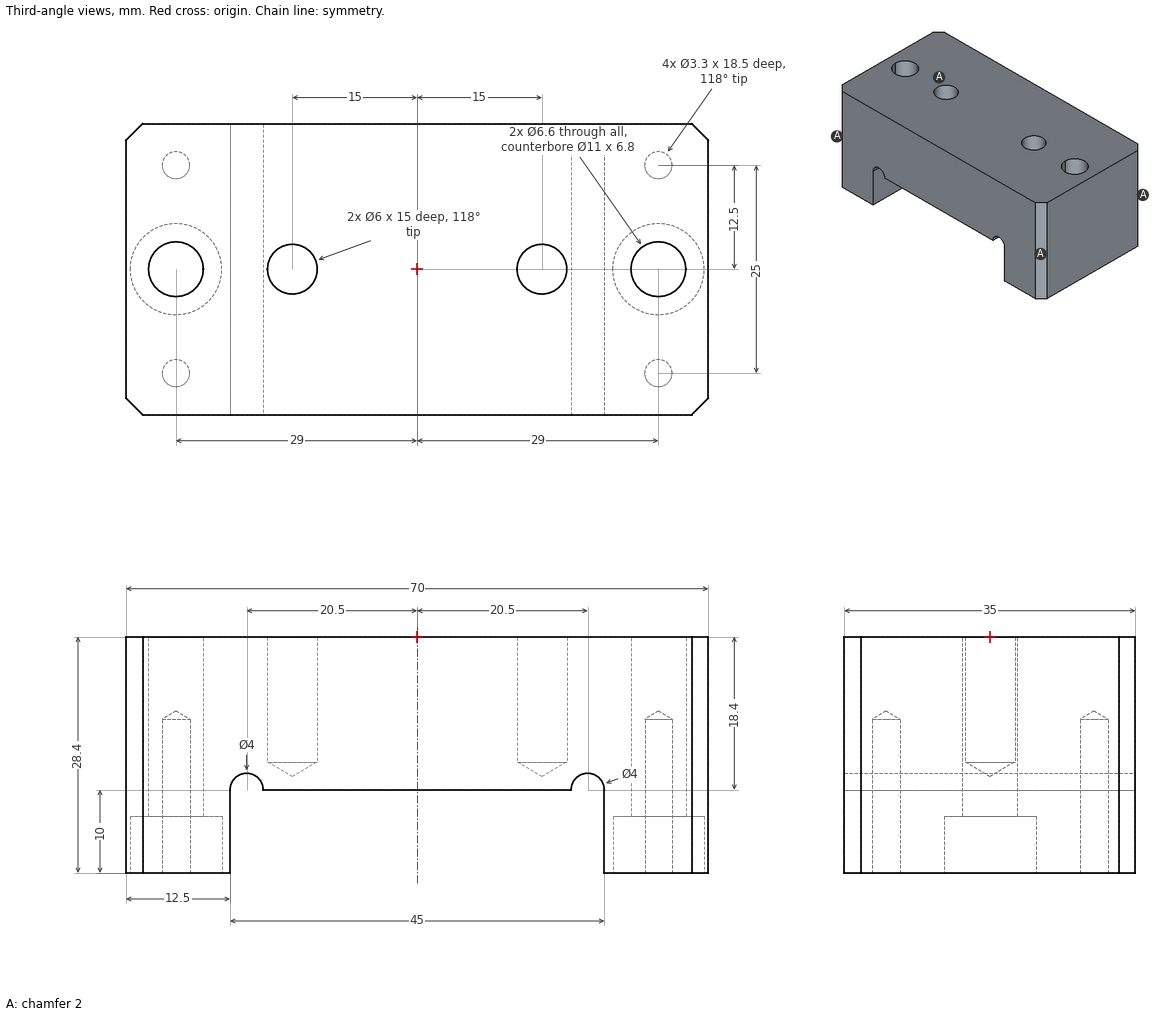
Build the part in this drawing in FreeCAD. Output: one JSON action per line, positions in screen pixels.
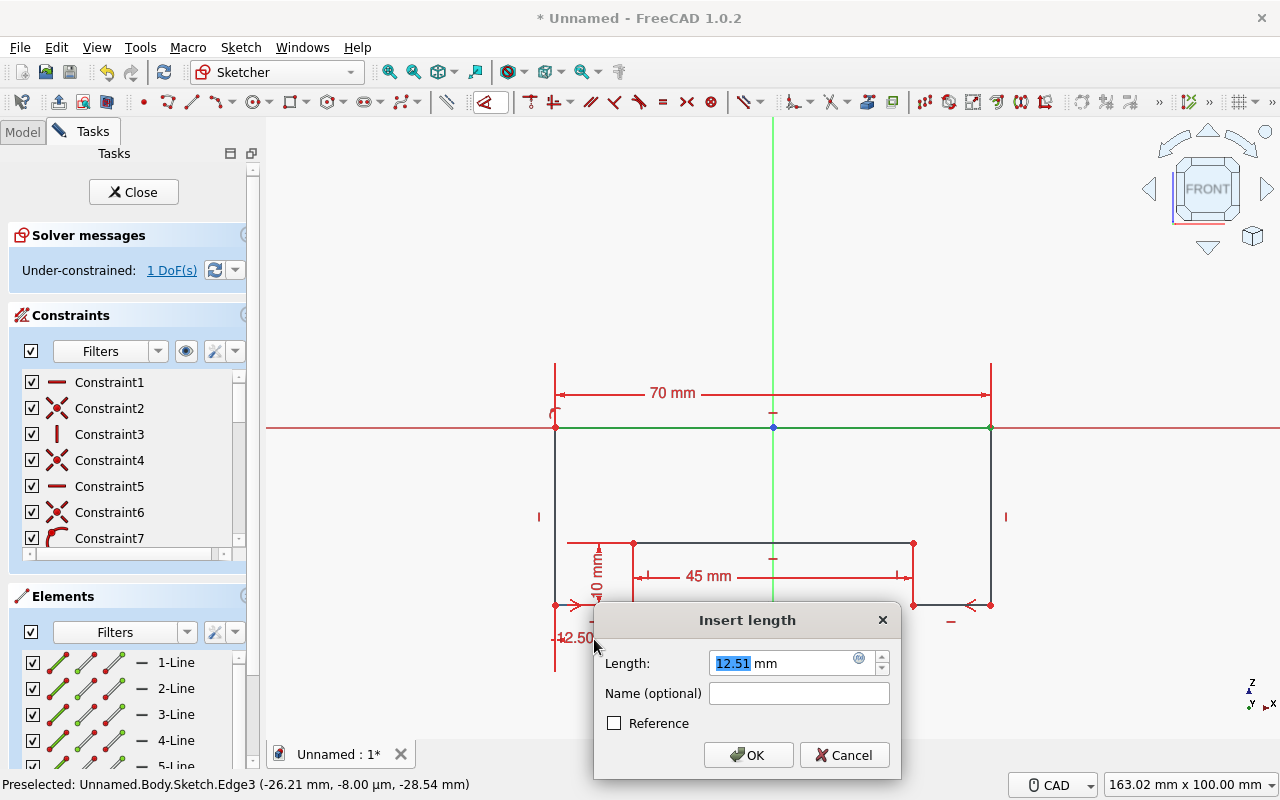
{"action": "type", "text": "12.5"}
{"action": "key", "text": "Return"}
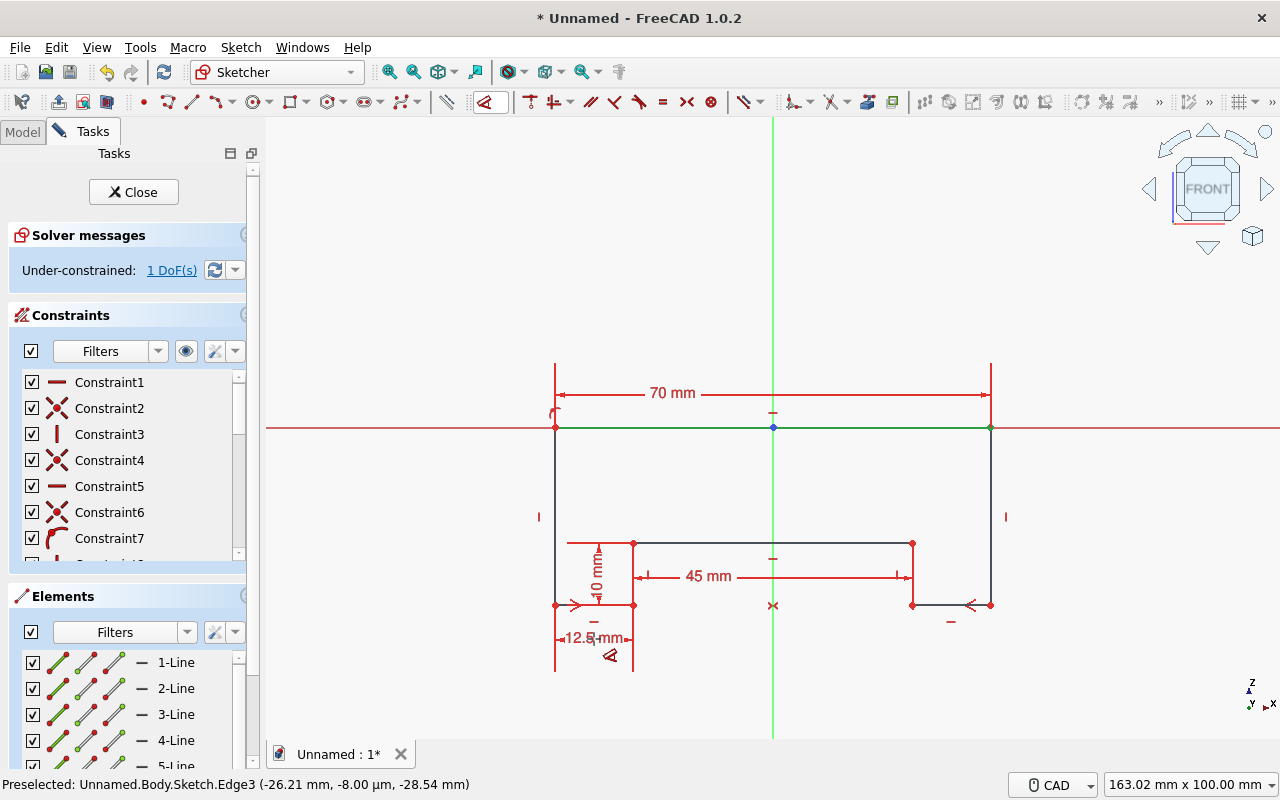
{"action": "left_click", "coordinate": [555, 552]}
{"action": "left_click", "coordinate": [521, 517]}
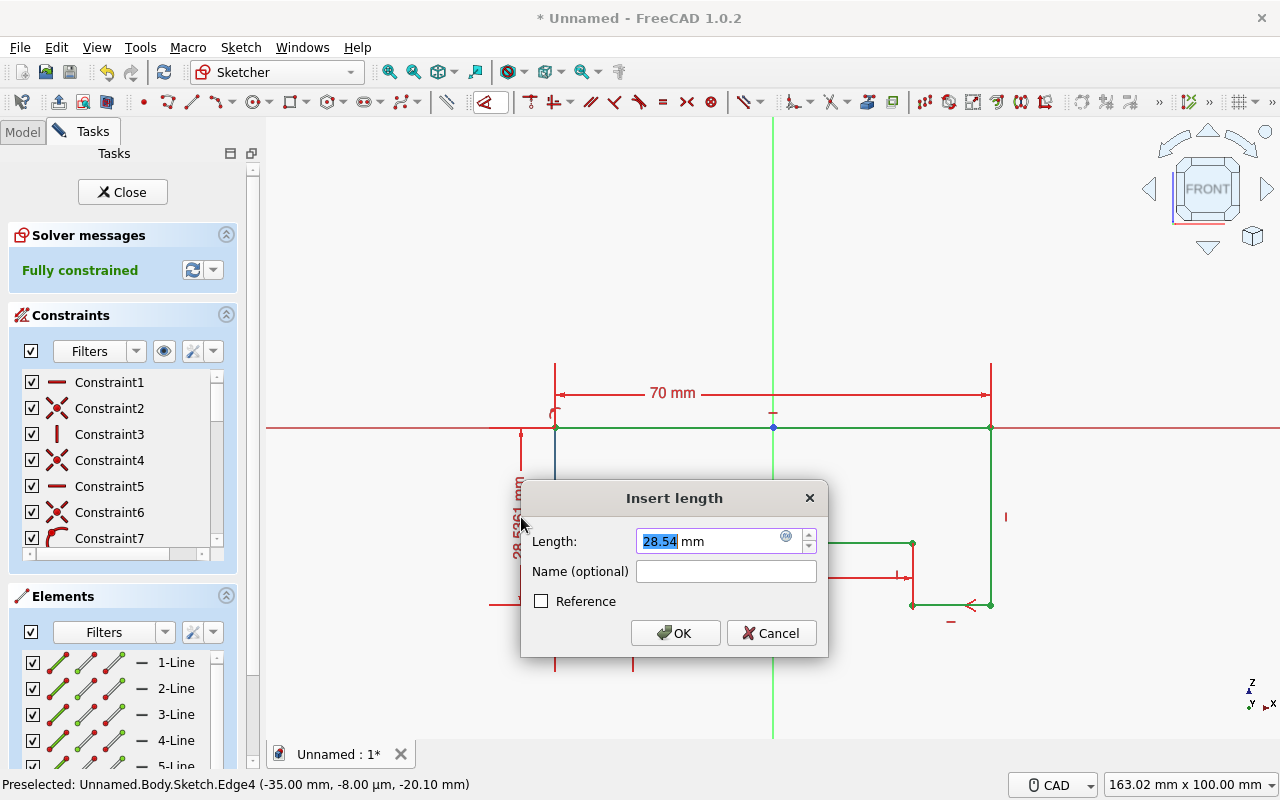
{"action": "type", "text": "28.4"}
{"action": "key", "text": "Return"}
{"action": "key", "text": "Escape"}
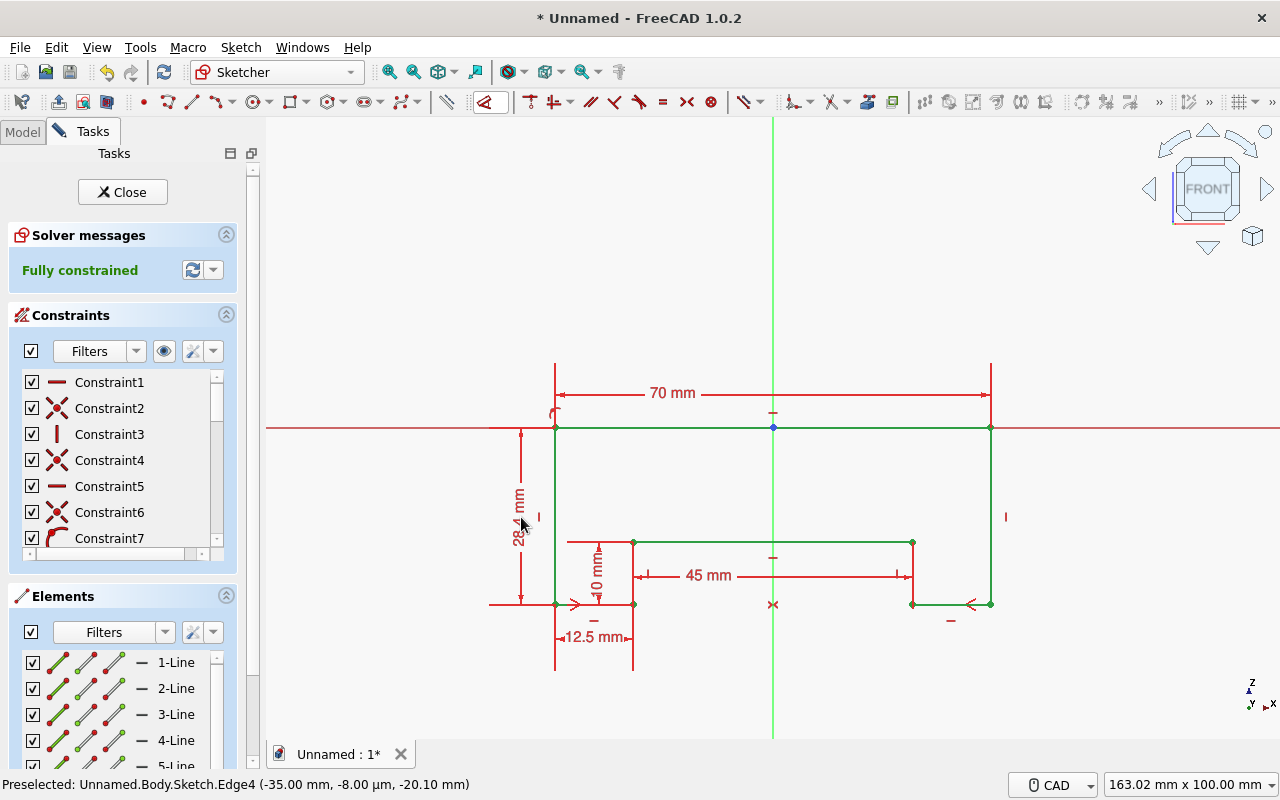
{"action": "left_click", "coordinate": [123, 192]}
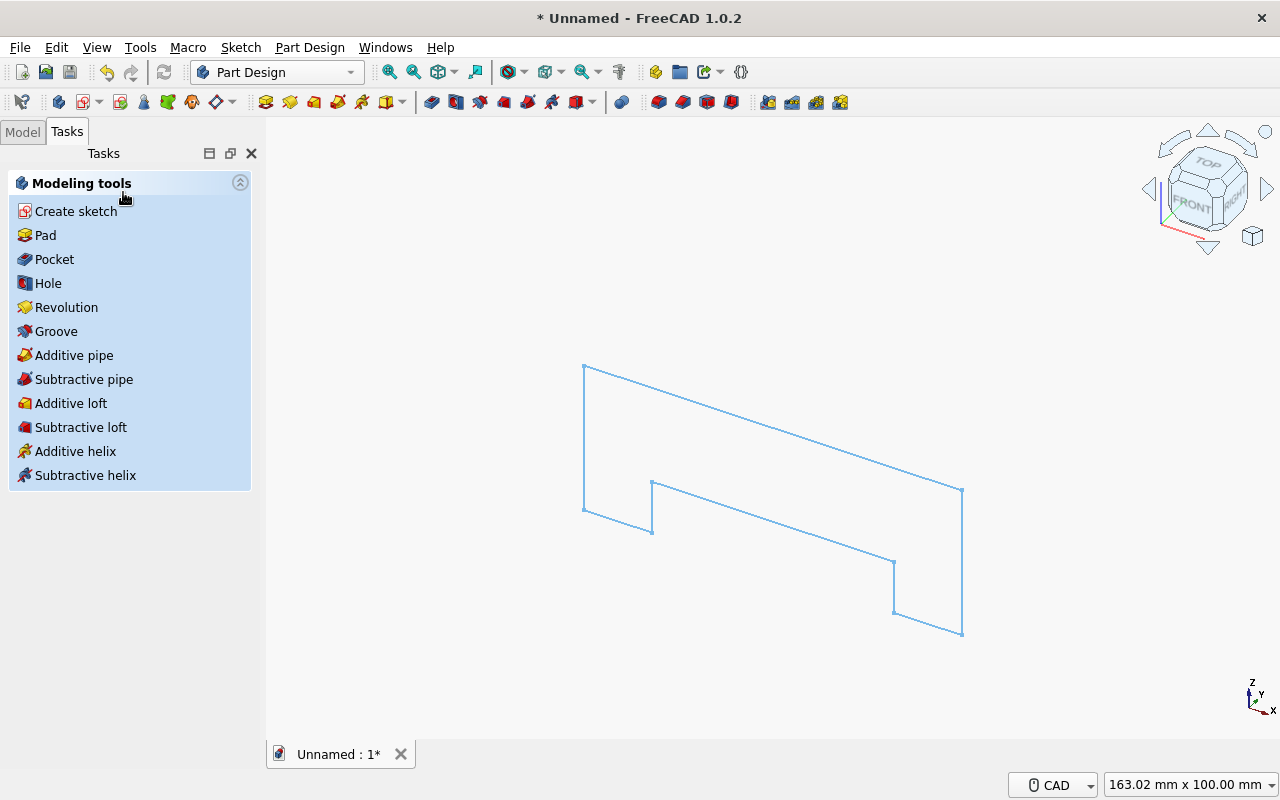
{"action": "left_click", "coordinate": [266, 102]}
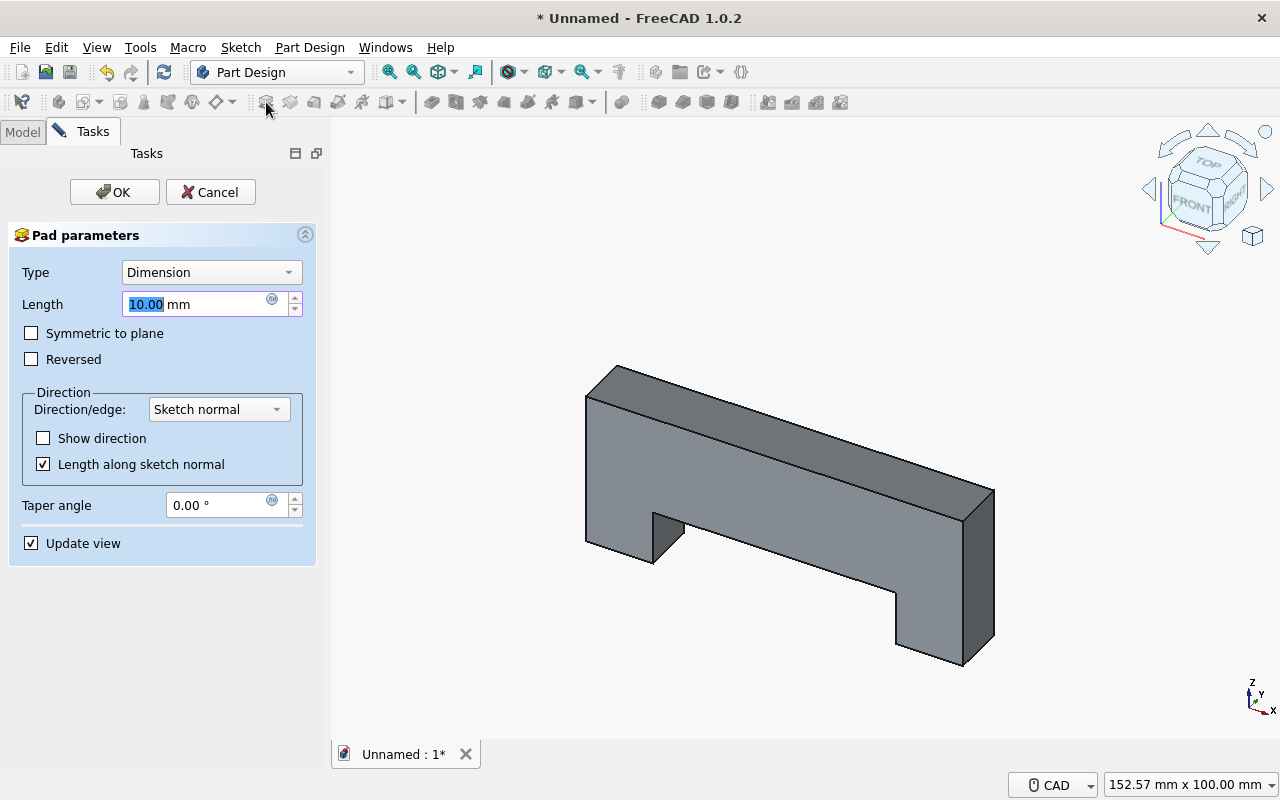
{"action": "type", "text": "35"}
{"action": "key", "text": "Tab"}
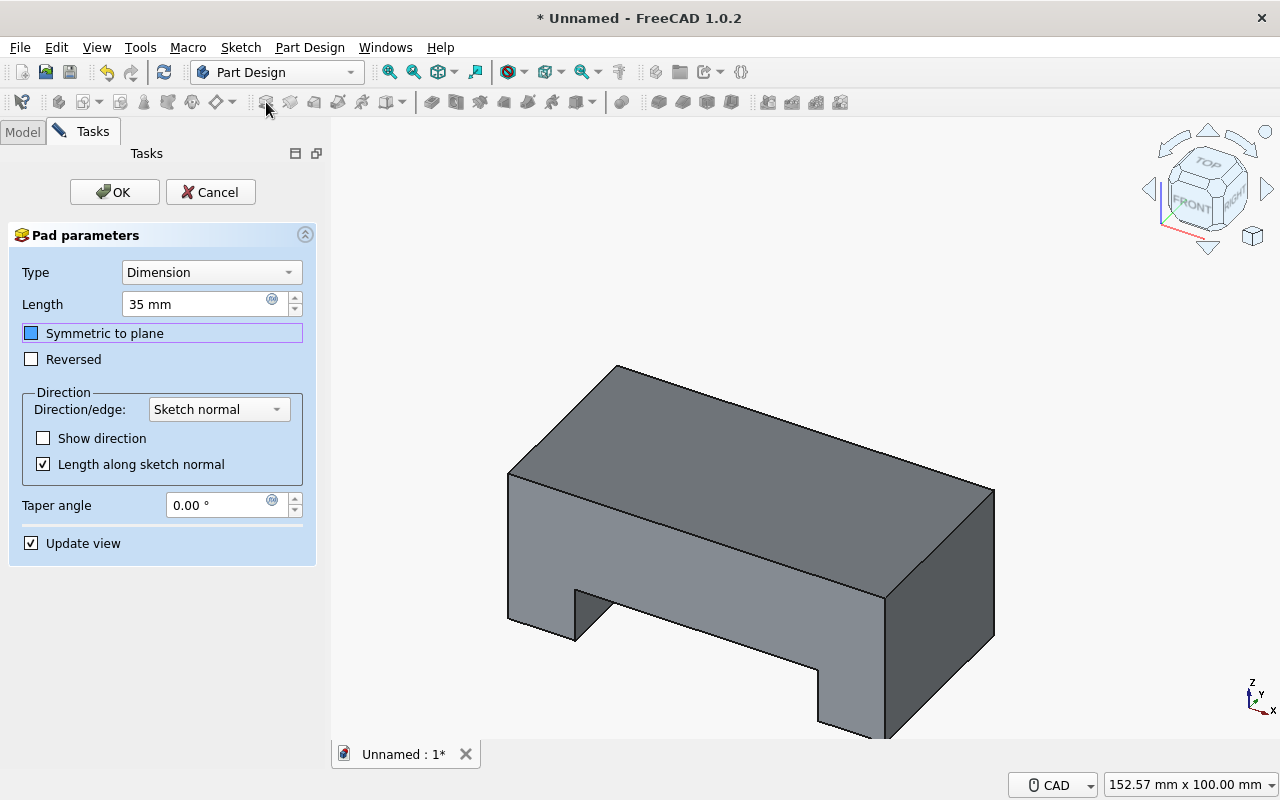
{"action": "left_click", "coordinate": [30, 333]}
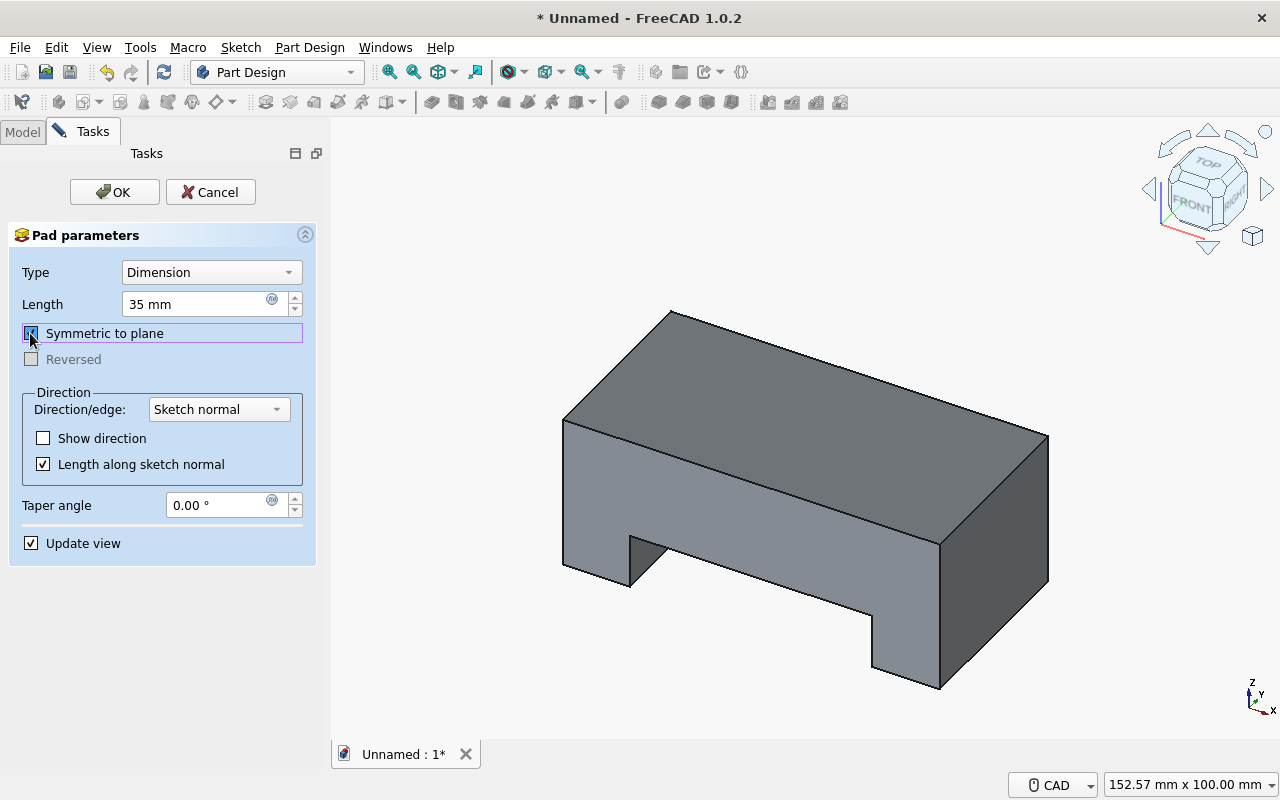
{"action": "left_click", "coordinate": [115, 192]}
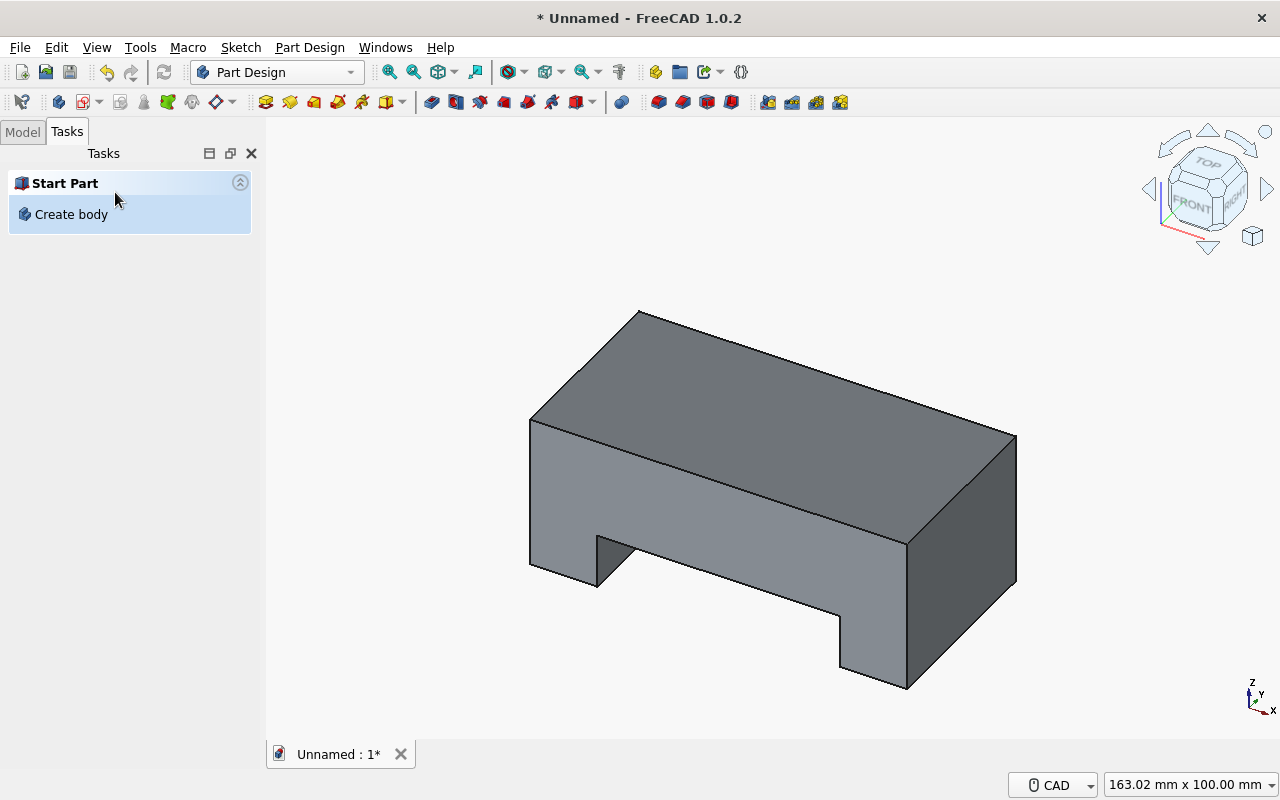
{"action": "key", "text": "4"}